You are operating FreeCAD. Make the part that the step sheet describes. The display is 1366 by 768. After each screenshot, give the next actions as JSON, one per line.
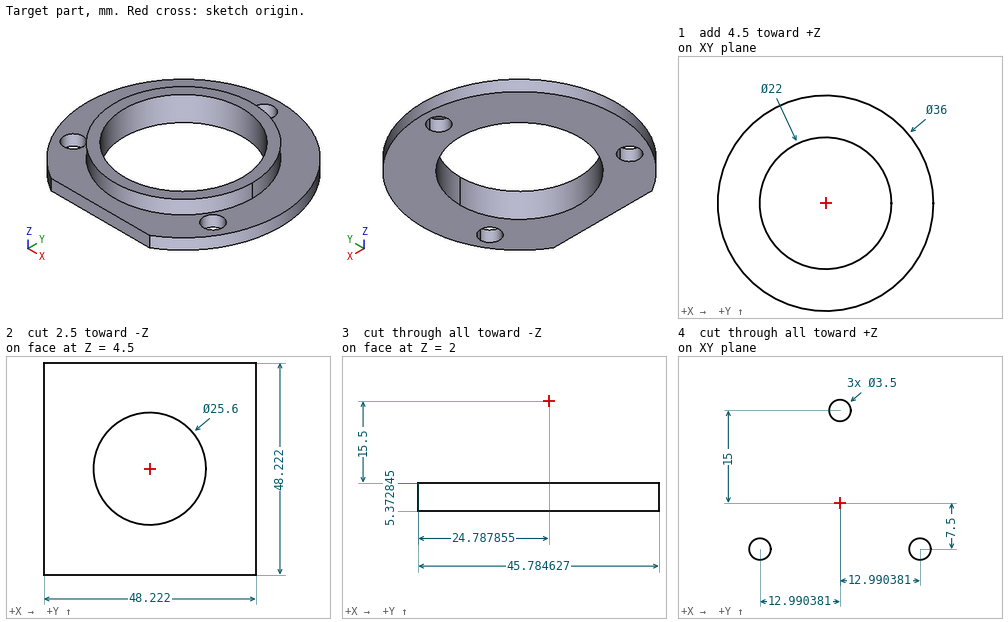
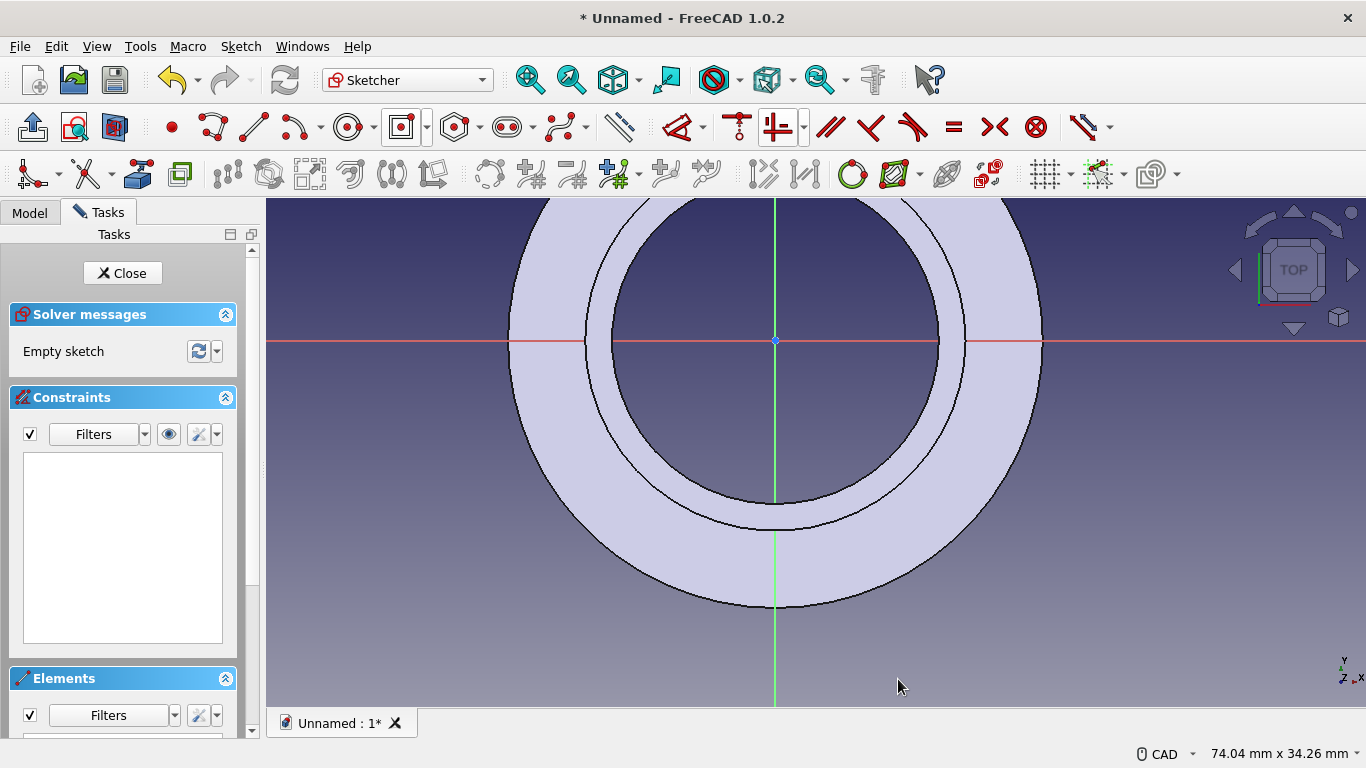
{"action": "left_click", "coordinate": [426, 128]}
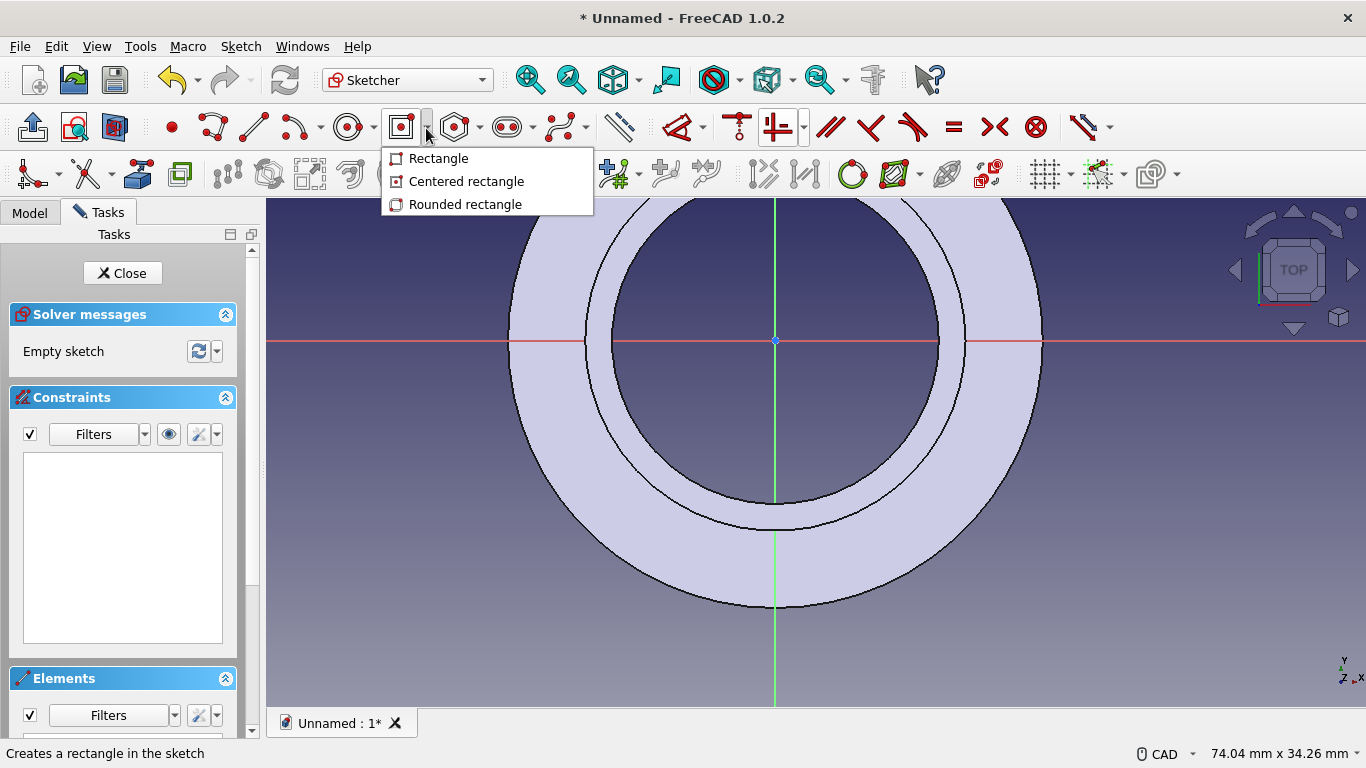
{"action": "left_click", "coordinate": [488, 158]}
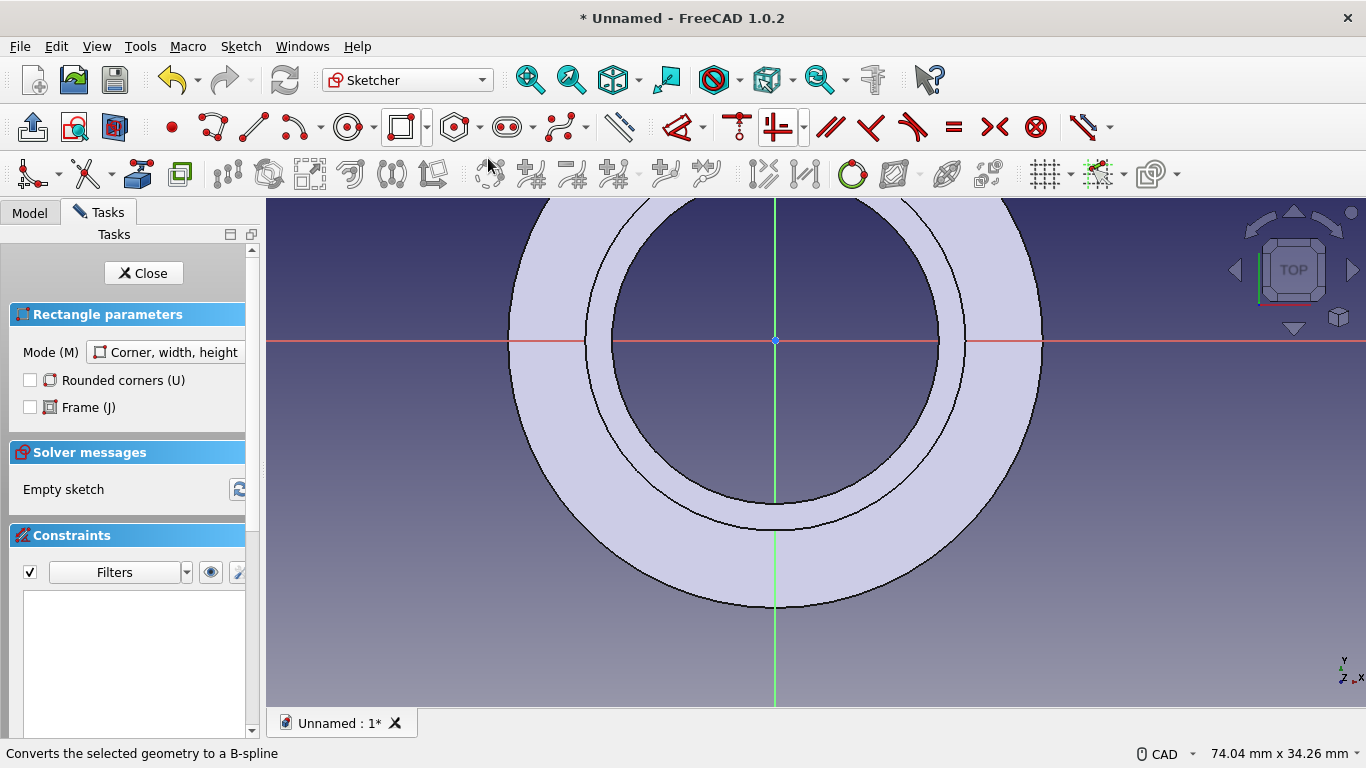
{"action": "left_click", "coordinate": [407, 571]}
{"action": "left_click", "coordinate": [1087, 651]}
{"action": "key", "text": "Escape"}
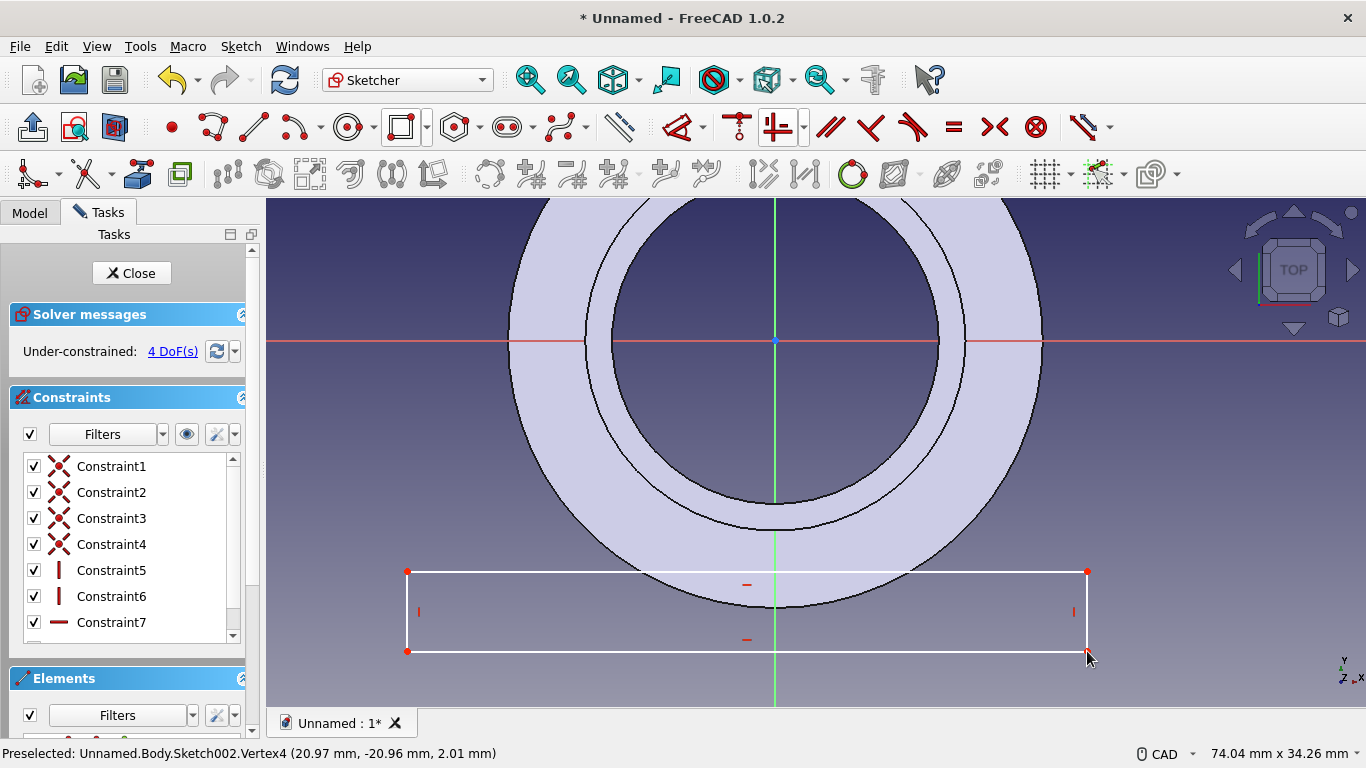
{"action": "left_click", "coordinate": [676, 128]}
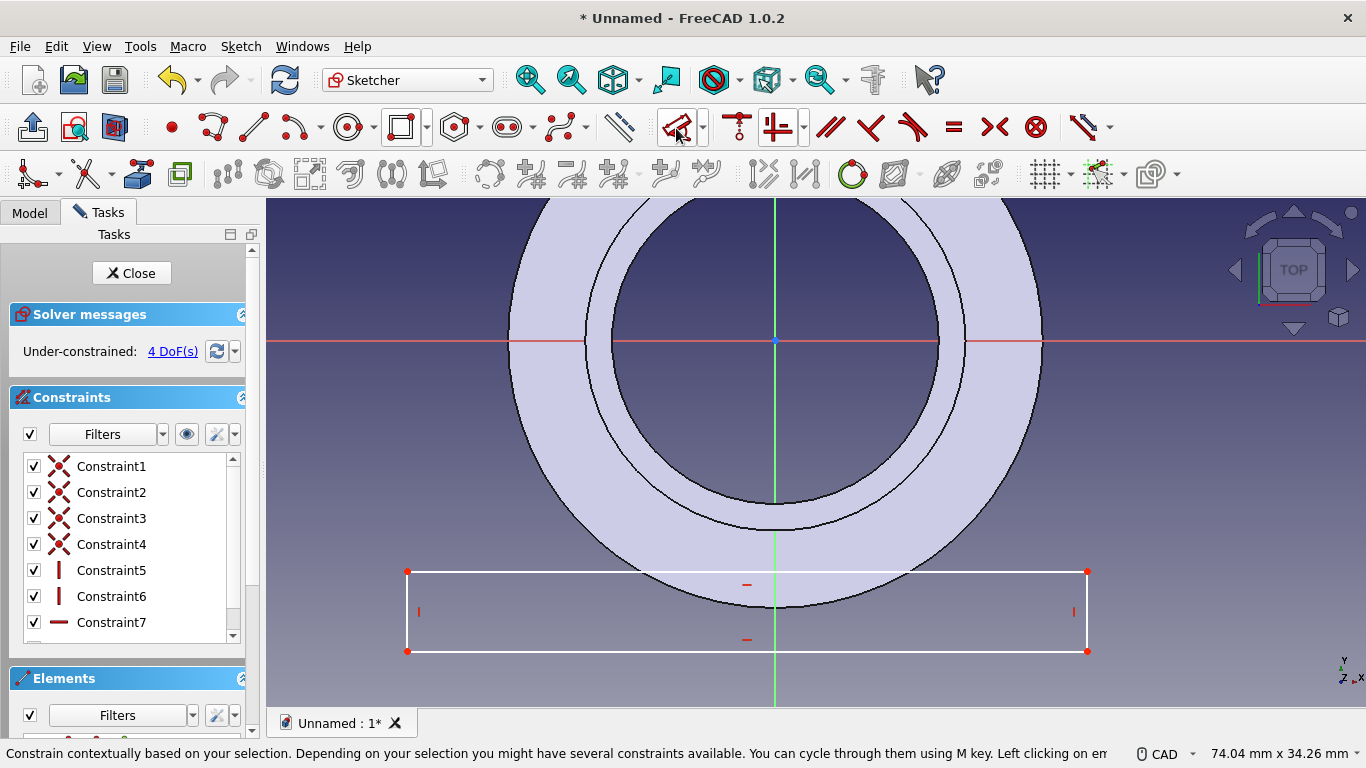
{"action": "left_click", "coordinate": [407, 572]}
{"action": "left_click", "coordinate": [373, 456]}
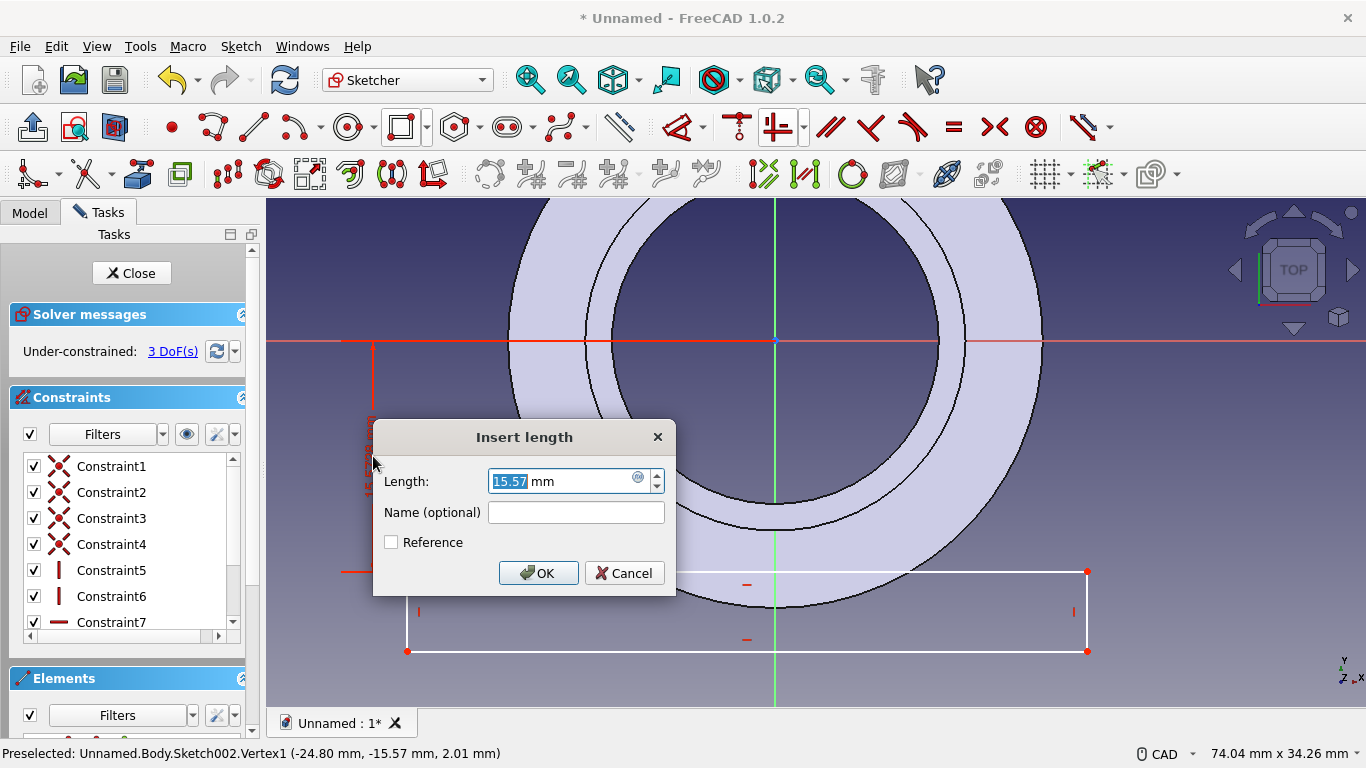
{"action": "type", "text": "15.5"}
{"action": "key", "text": "Return"}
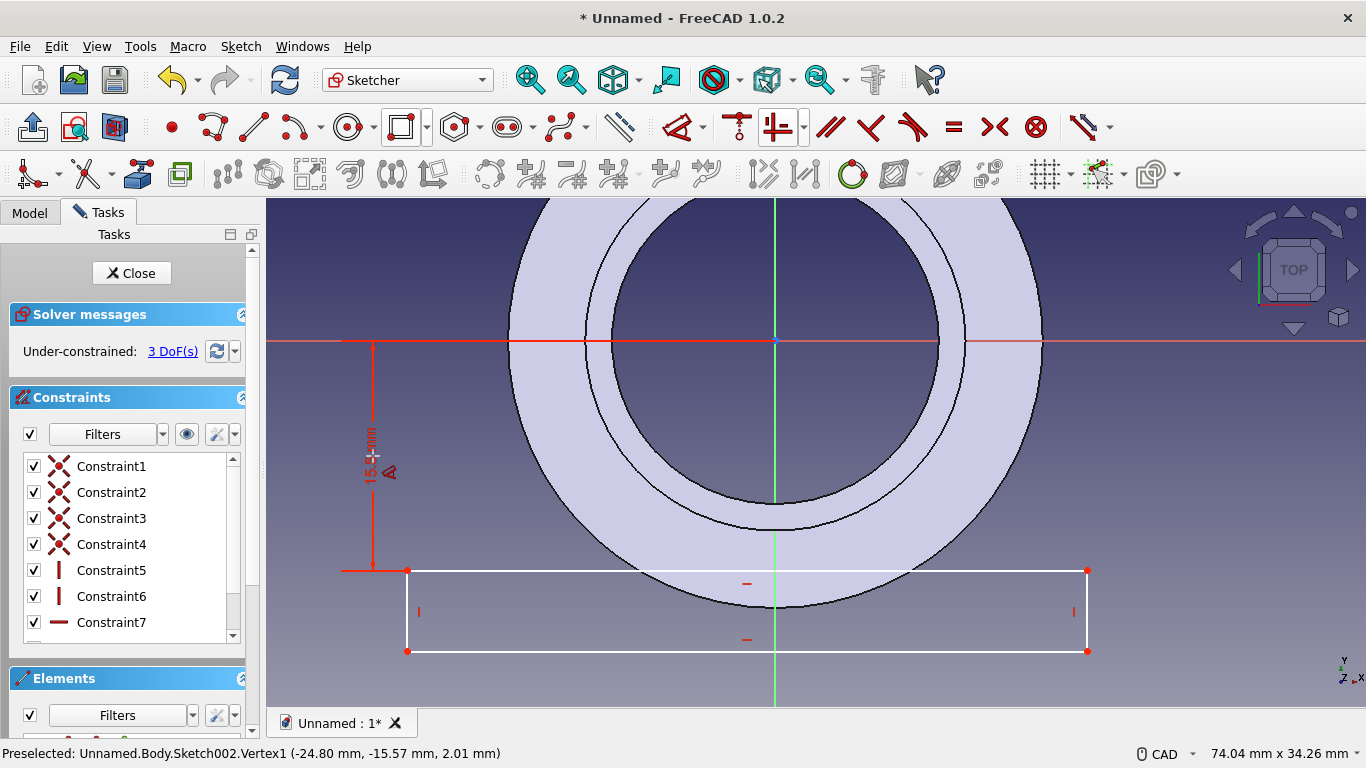
{"action": "left_click", "coordinate": [407, 595]}
{"action": "left_click", "coordinate": [373, 611]}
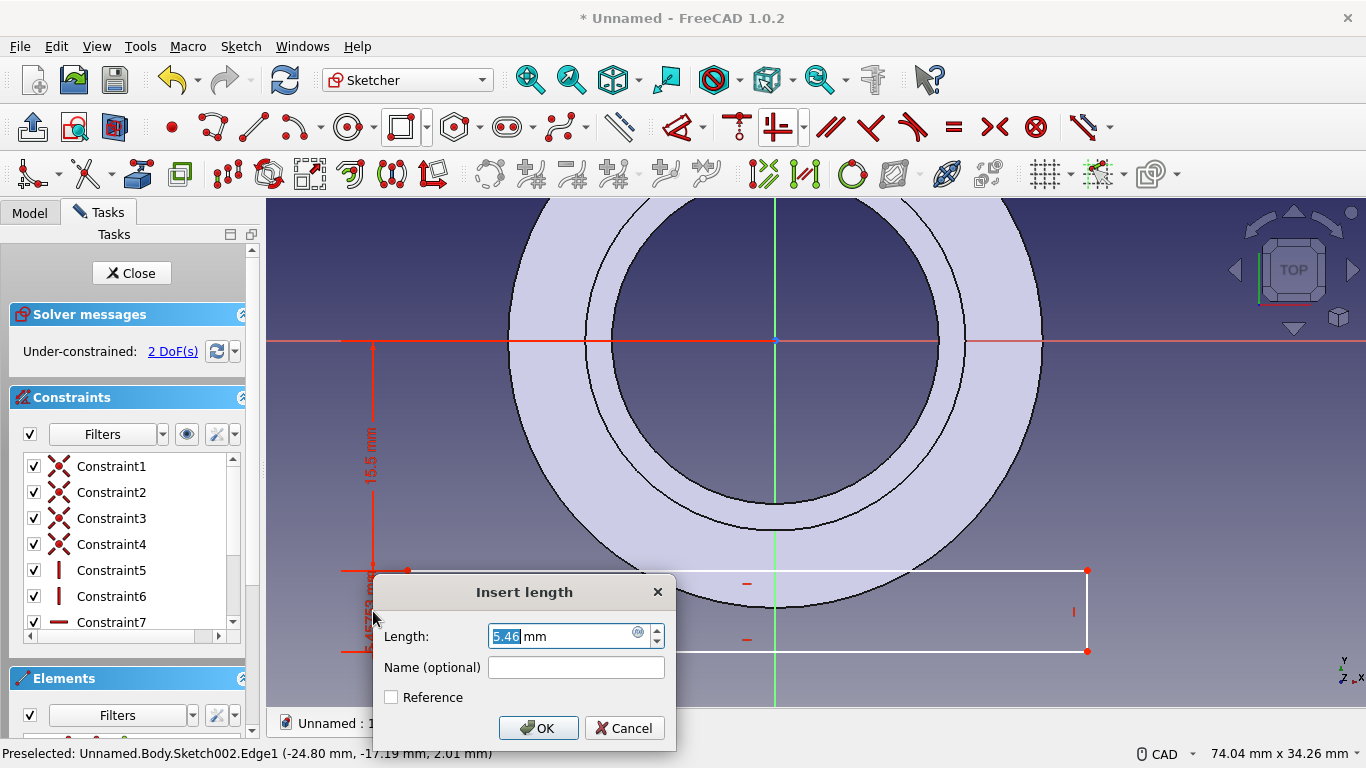
{"action": "type", "text": "5.372845"}
{"action": "key", "text": "Return"}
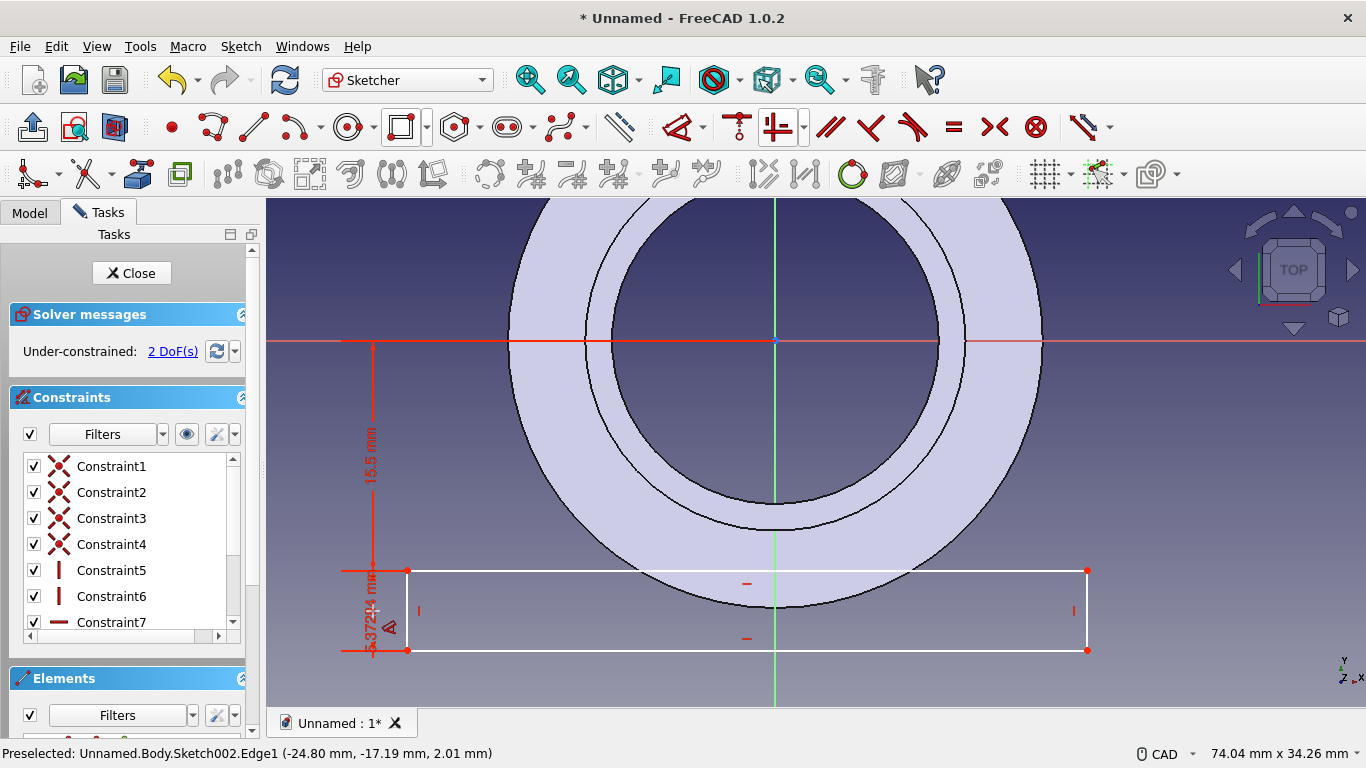
{"action": "left_click", "coordinate": [611, 651]}
{"action": "left_click", "coordinate": [747, 617]}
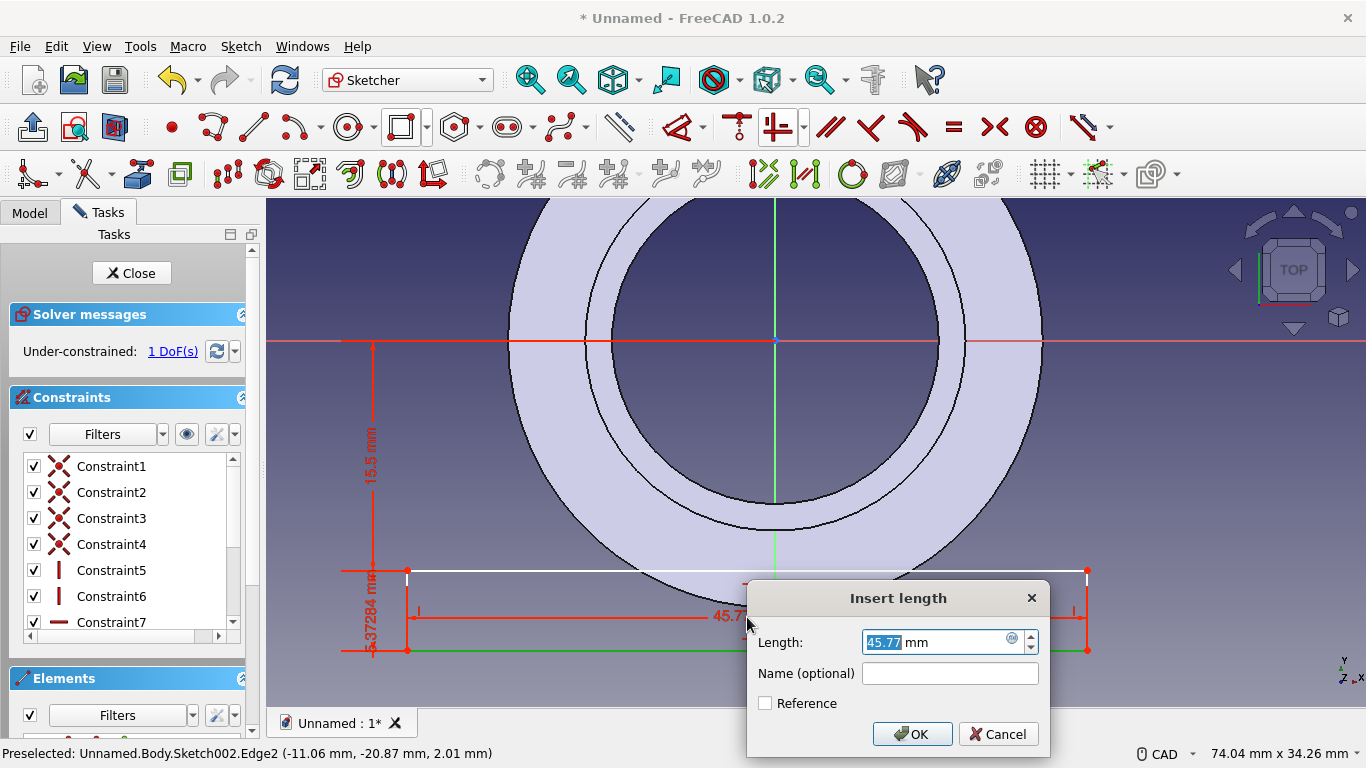
{"action": "type", "text": "45.784627"}
{"action": "key", "text": "Return"}